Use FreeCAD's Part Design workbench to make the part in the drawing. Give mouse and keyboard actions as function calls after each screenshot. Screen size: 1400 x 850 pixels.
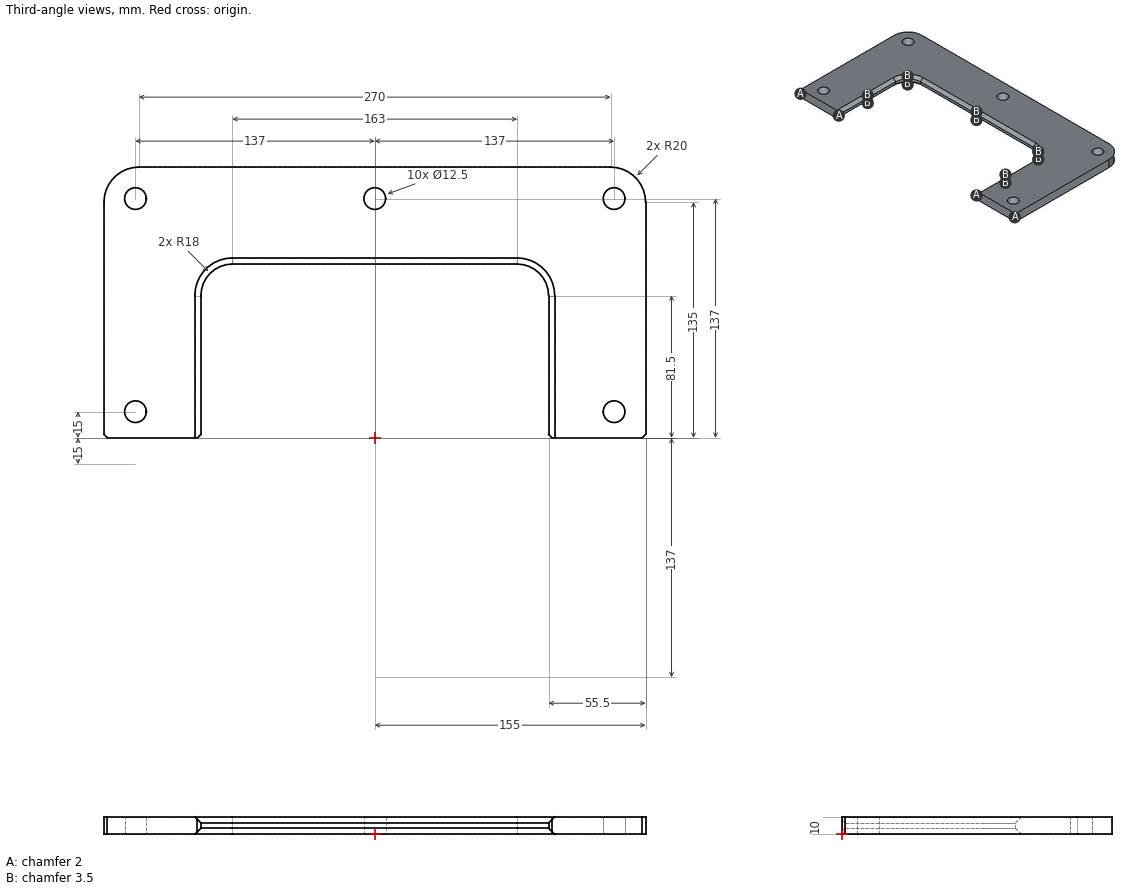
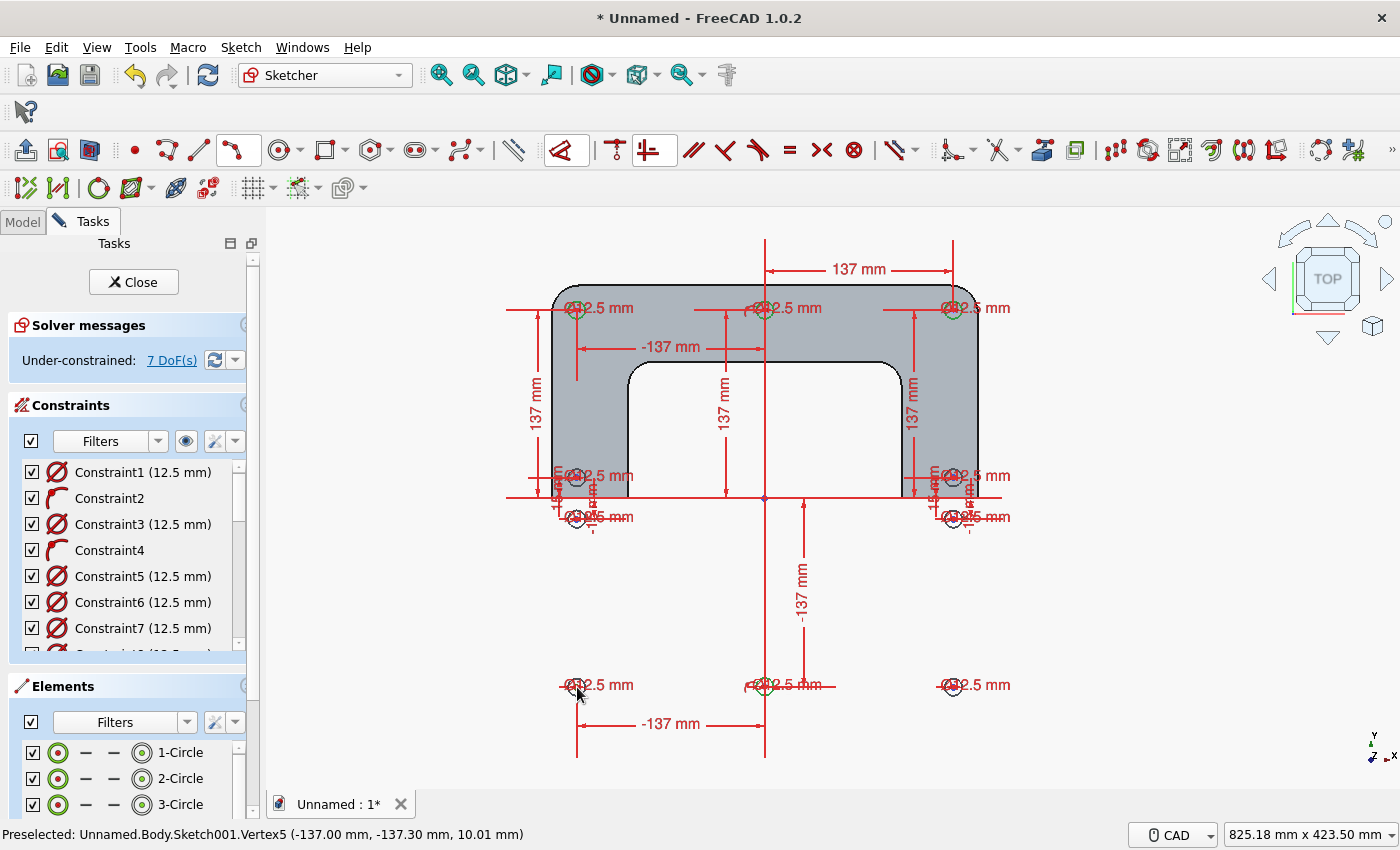
key(i)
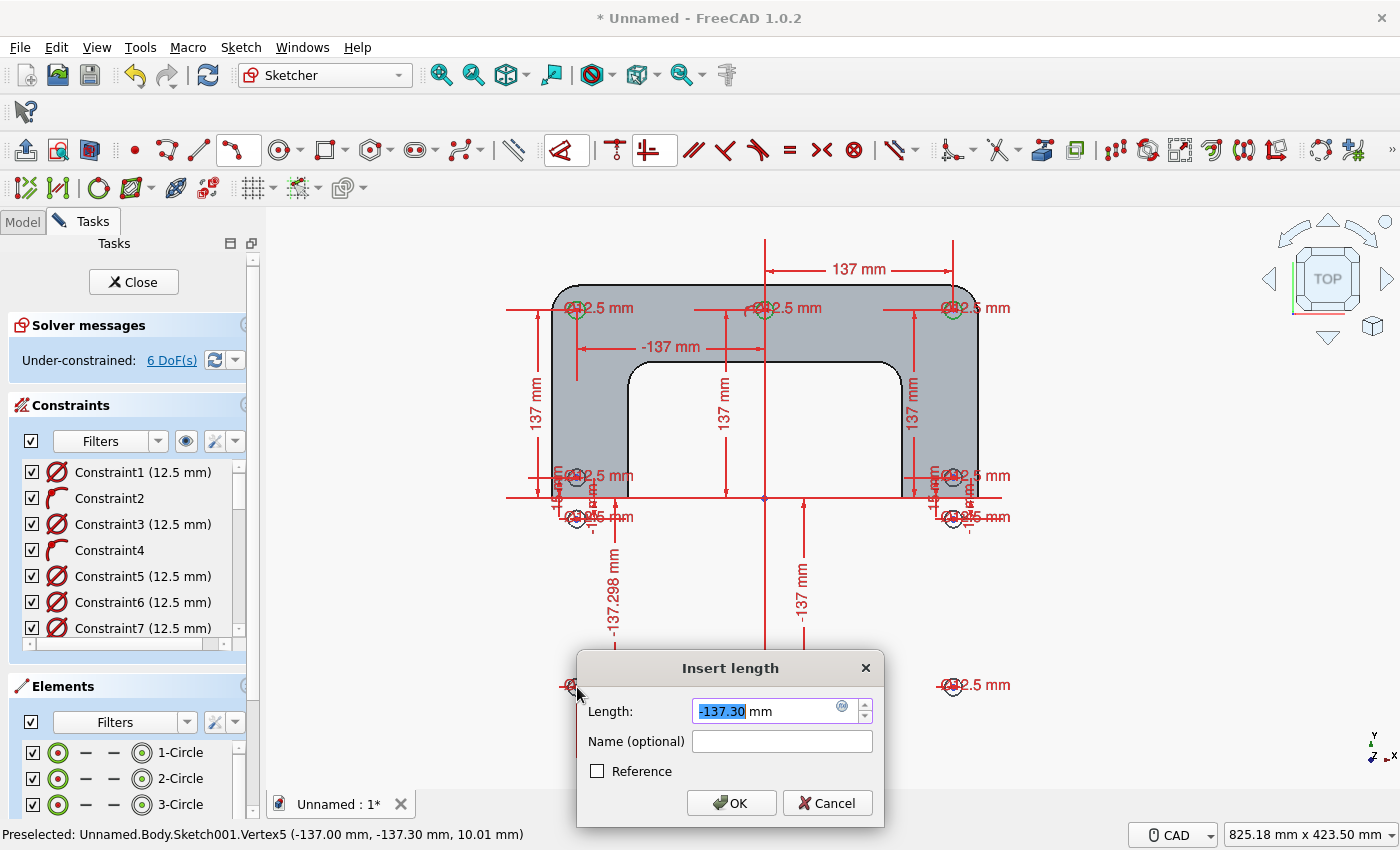
text(-137)
key(Return)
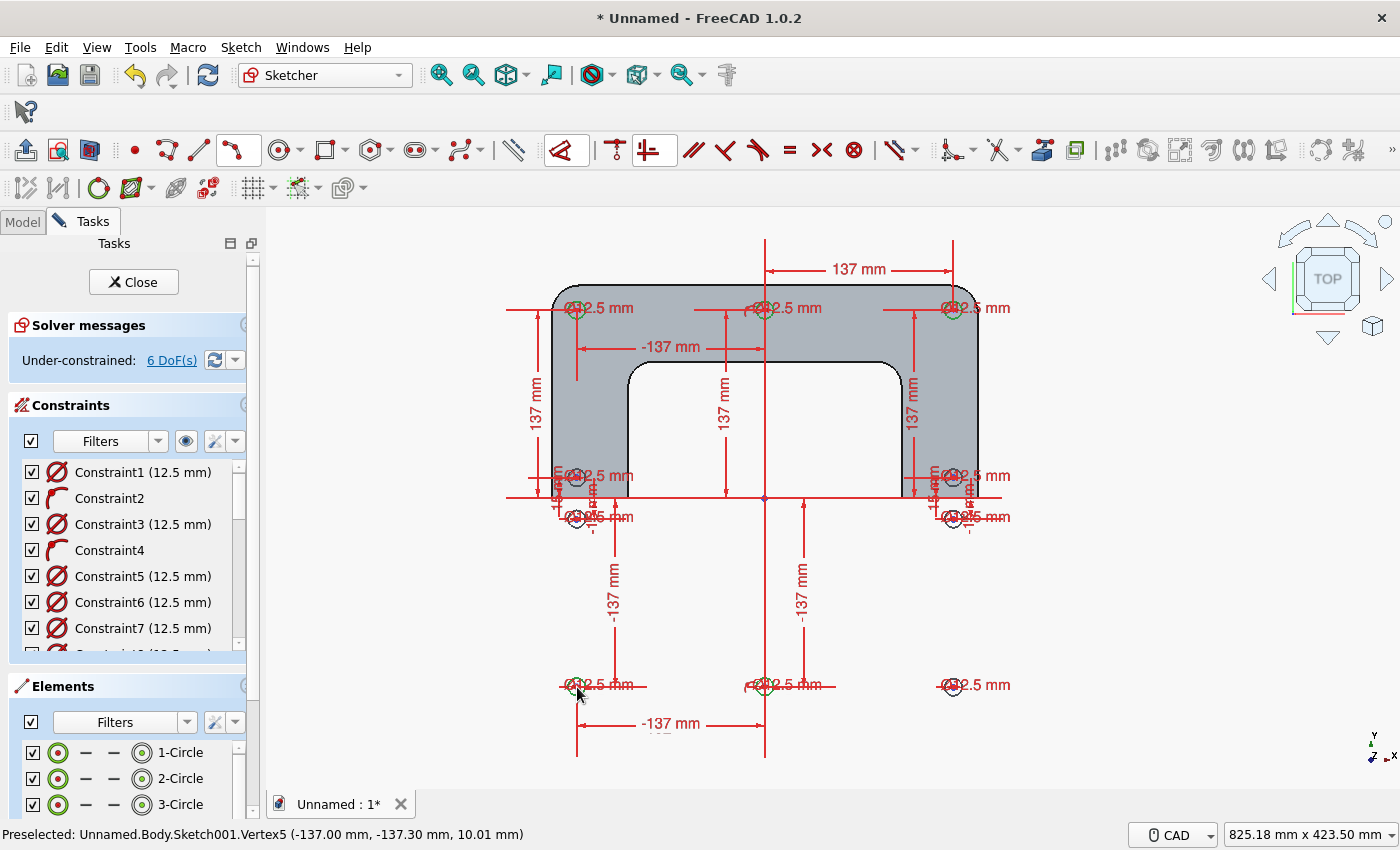
click(953, 687)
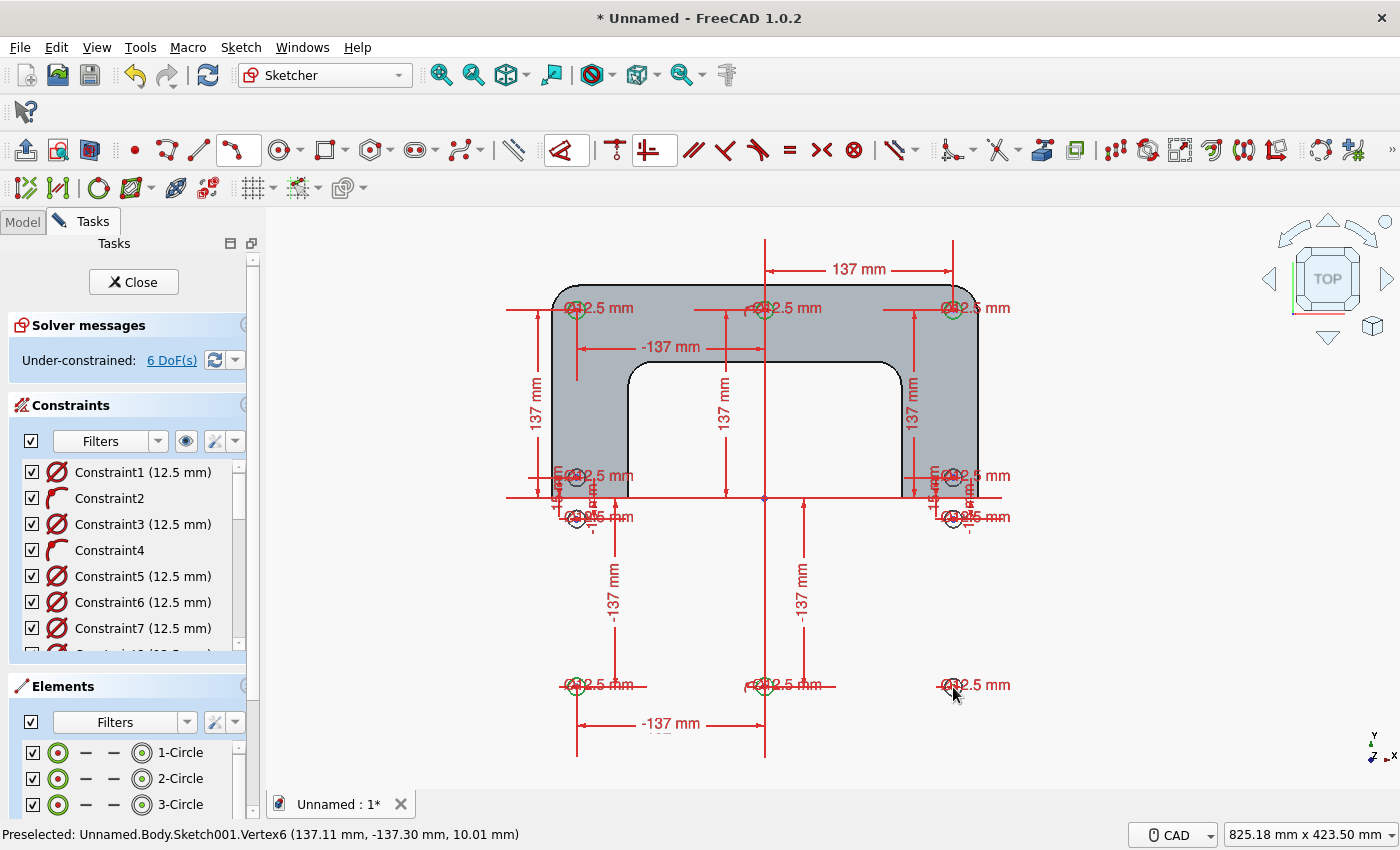
key(l)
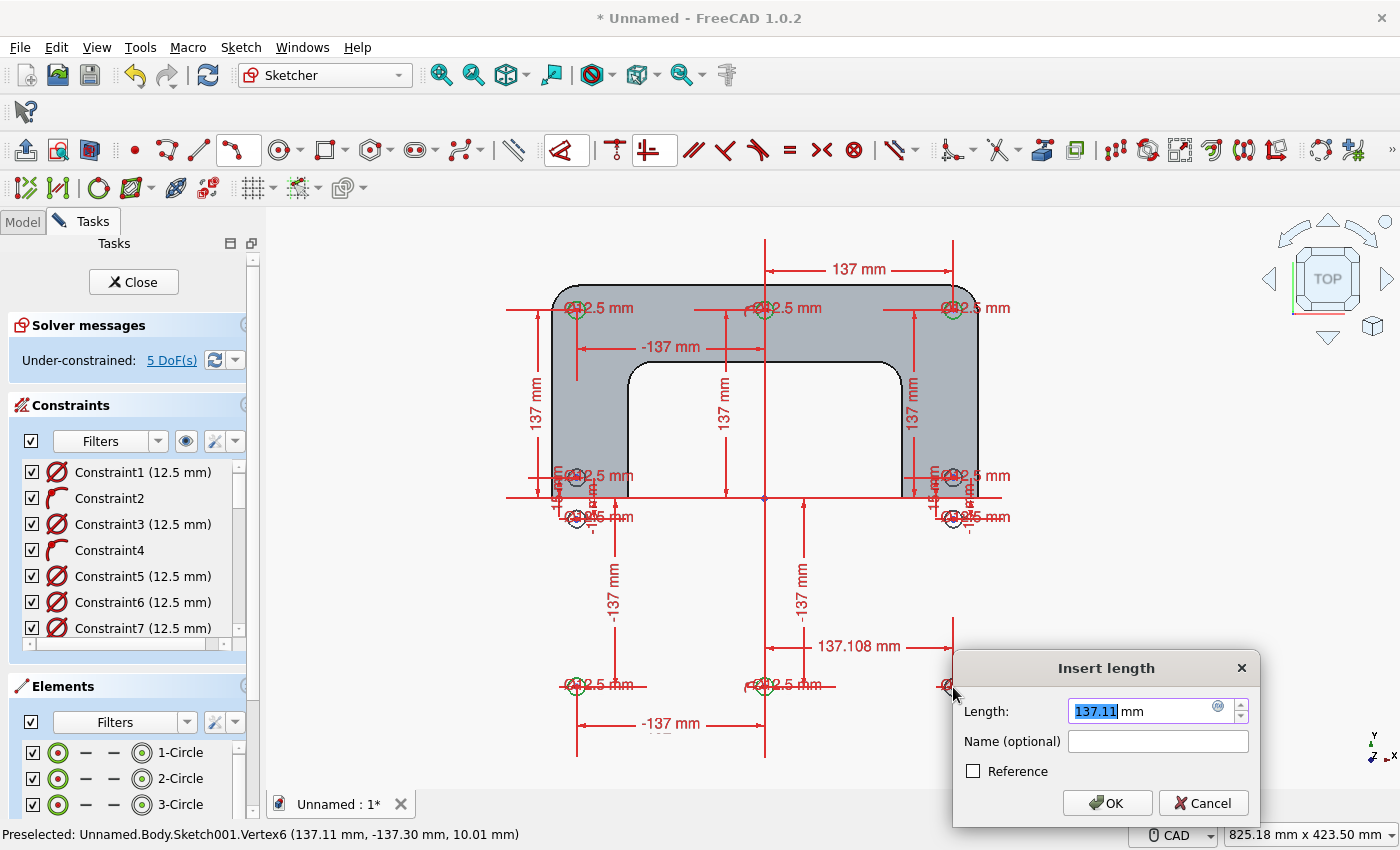
text(137)
key(Return)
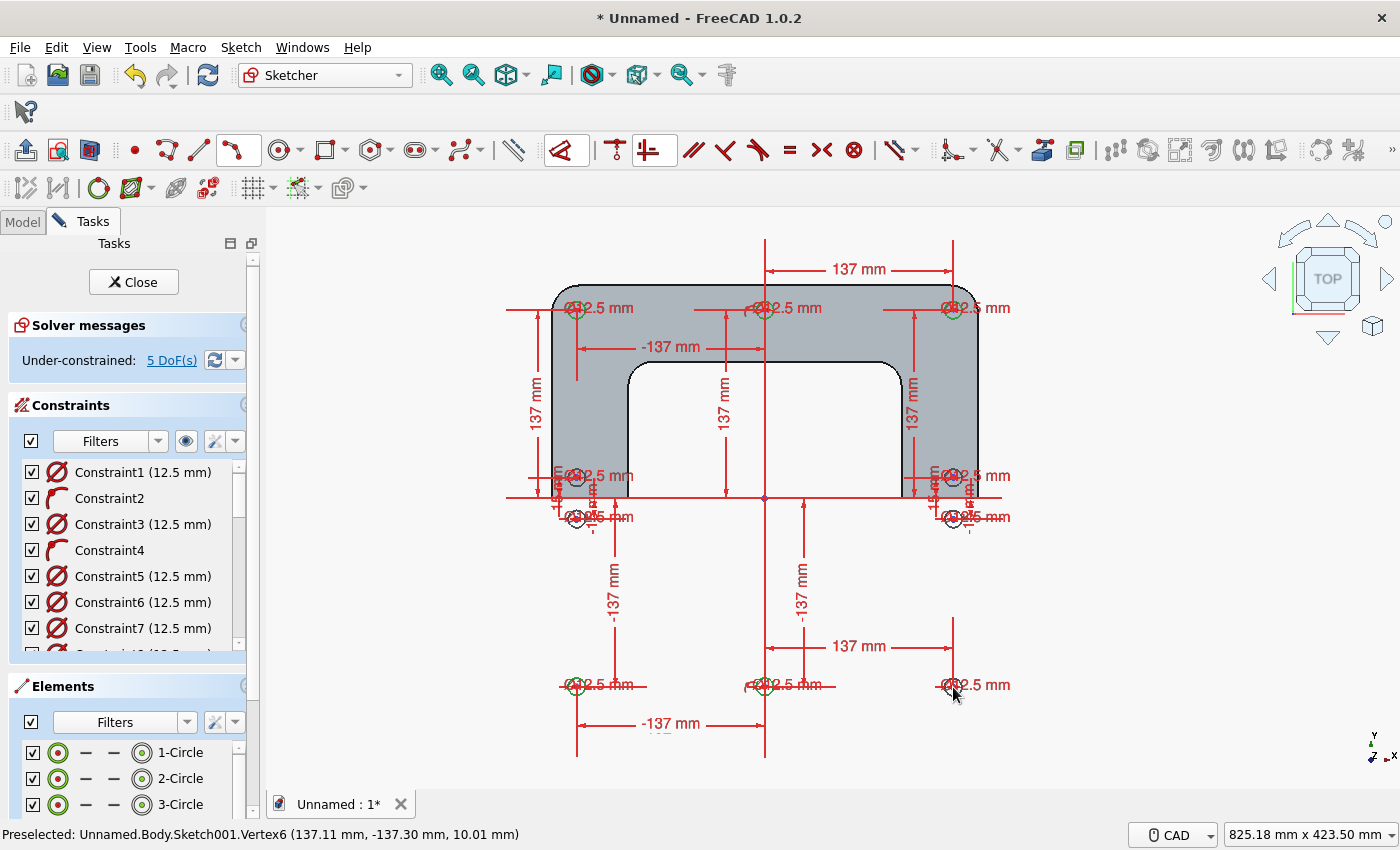
click(953, 687)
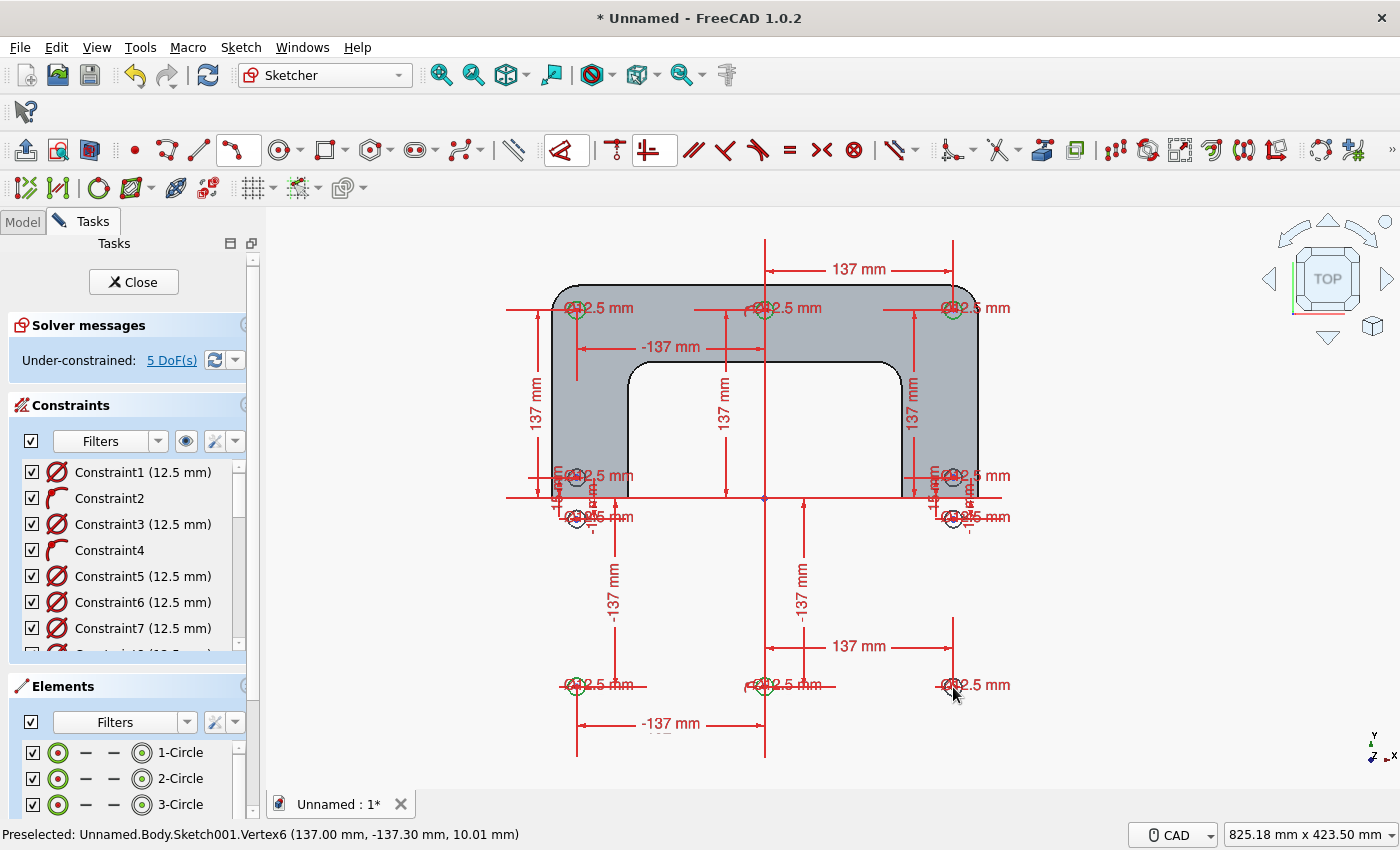
key(i)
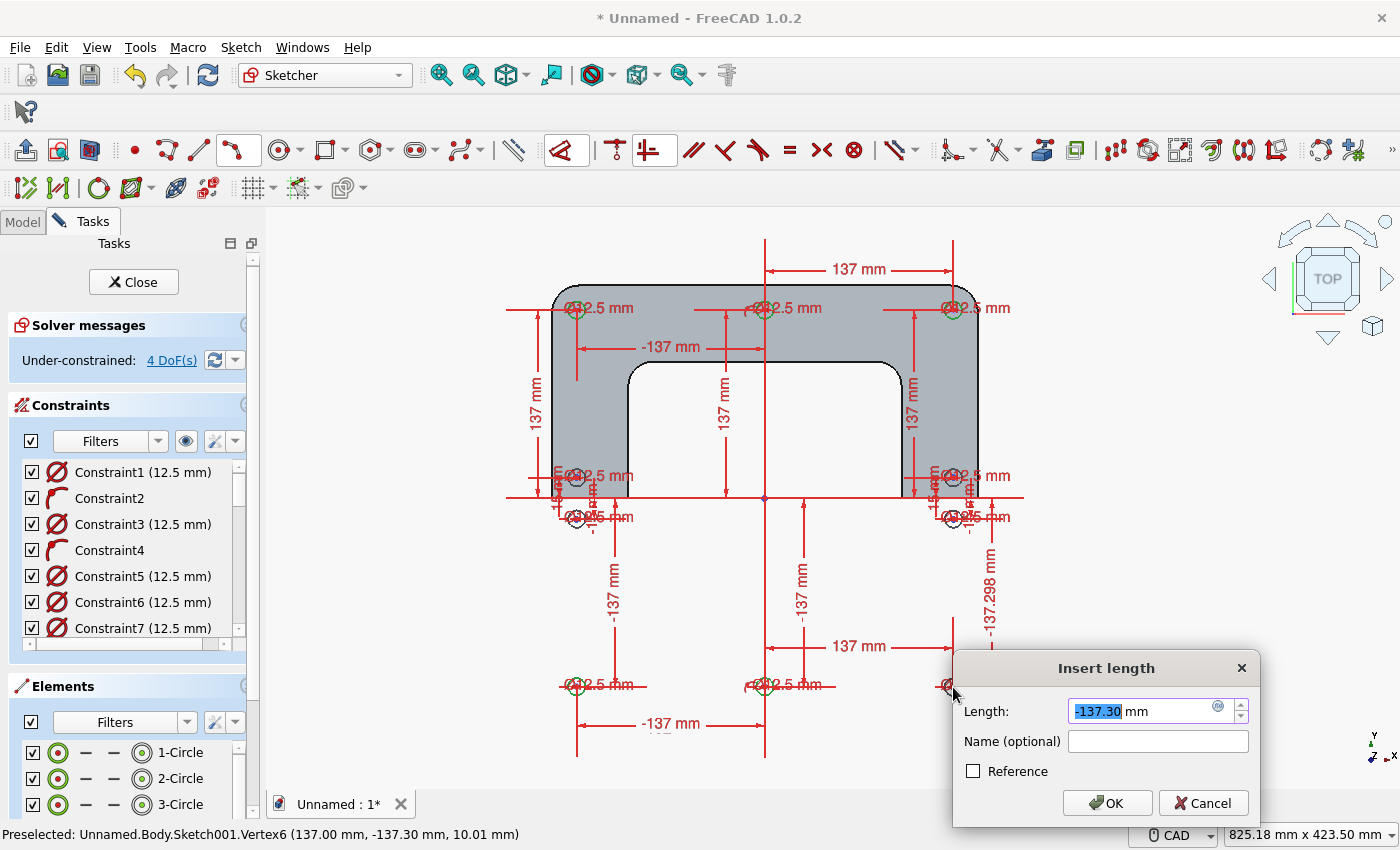
text(-137)
key(Return)